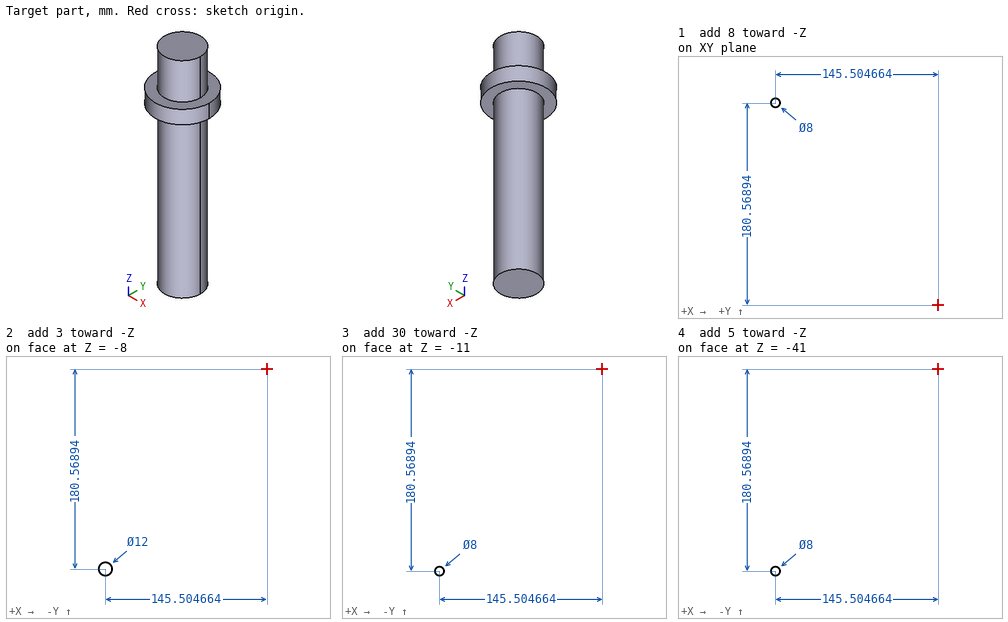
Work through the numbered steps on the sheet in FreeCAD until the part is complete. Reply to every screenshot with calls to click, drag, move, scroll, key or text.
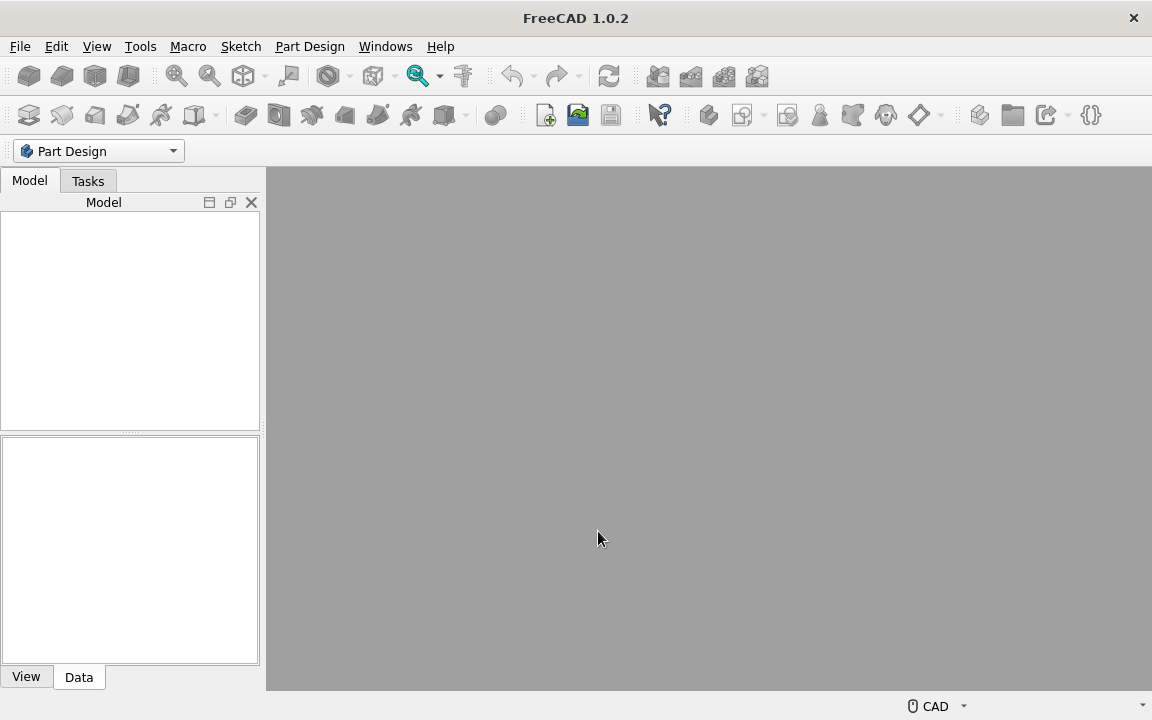
click(545, 116)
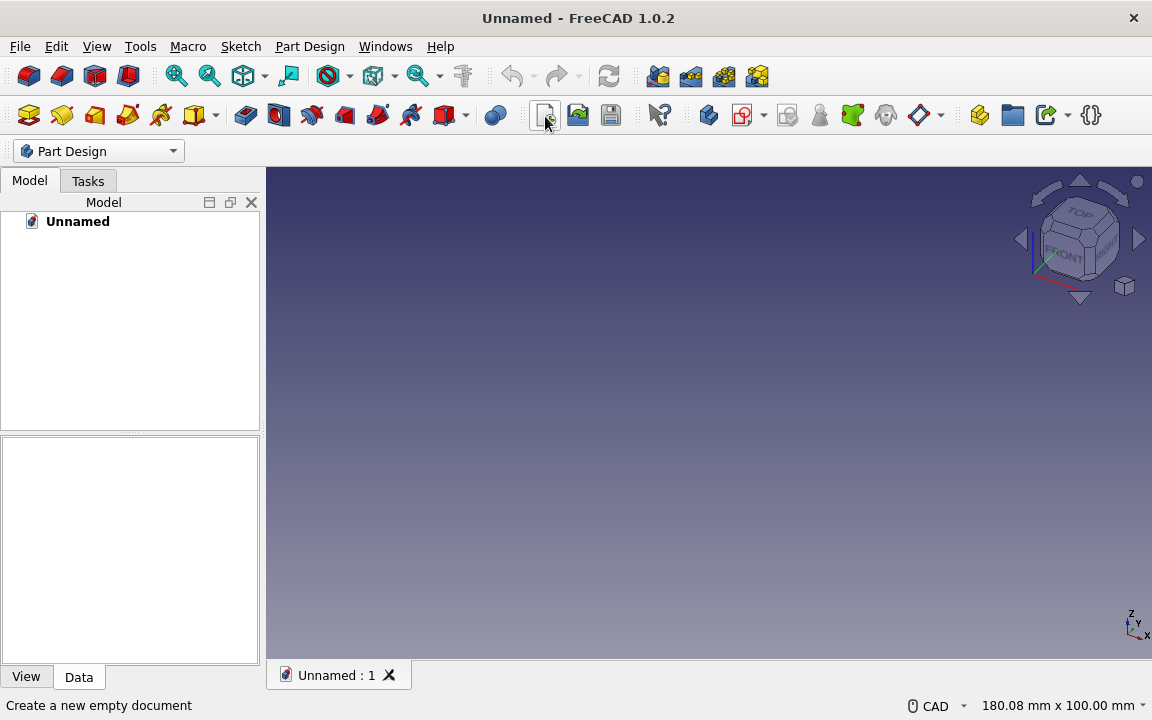
click(742, 116)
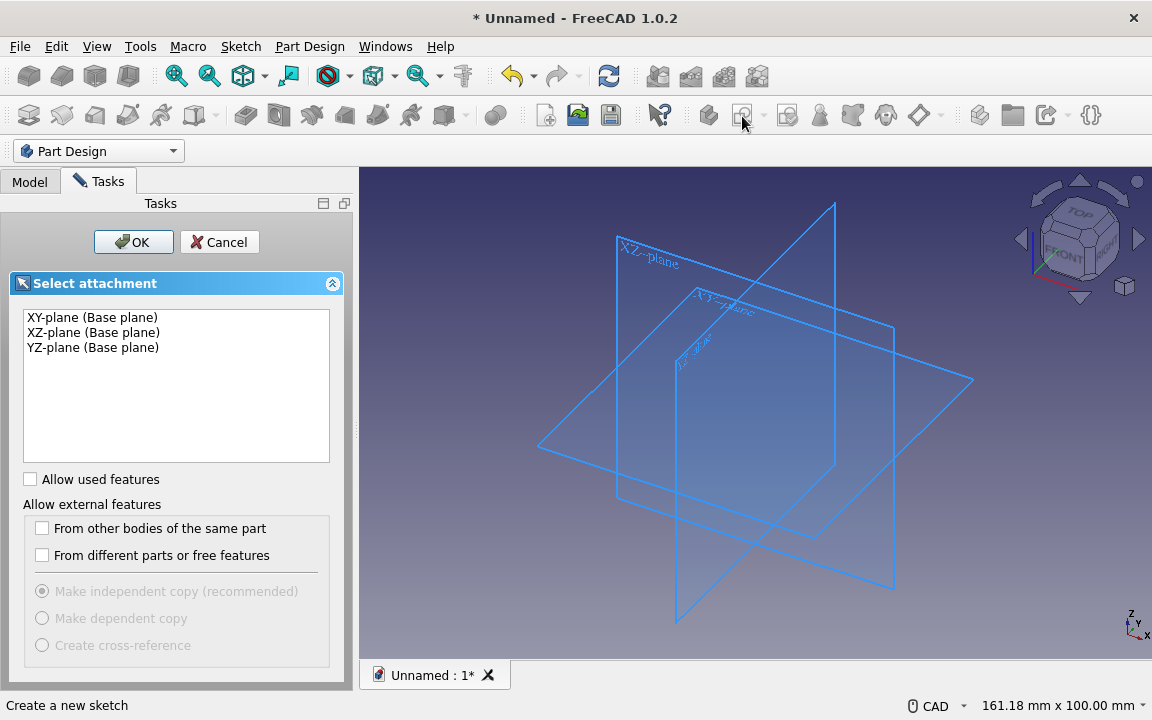
click(84, 318)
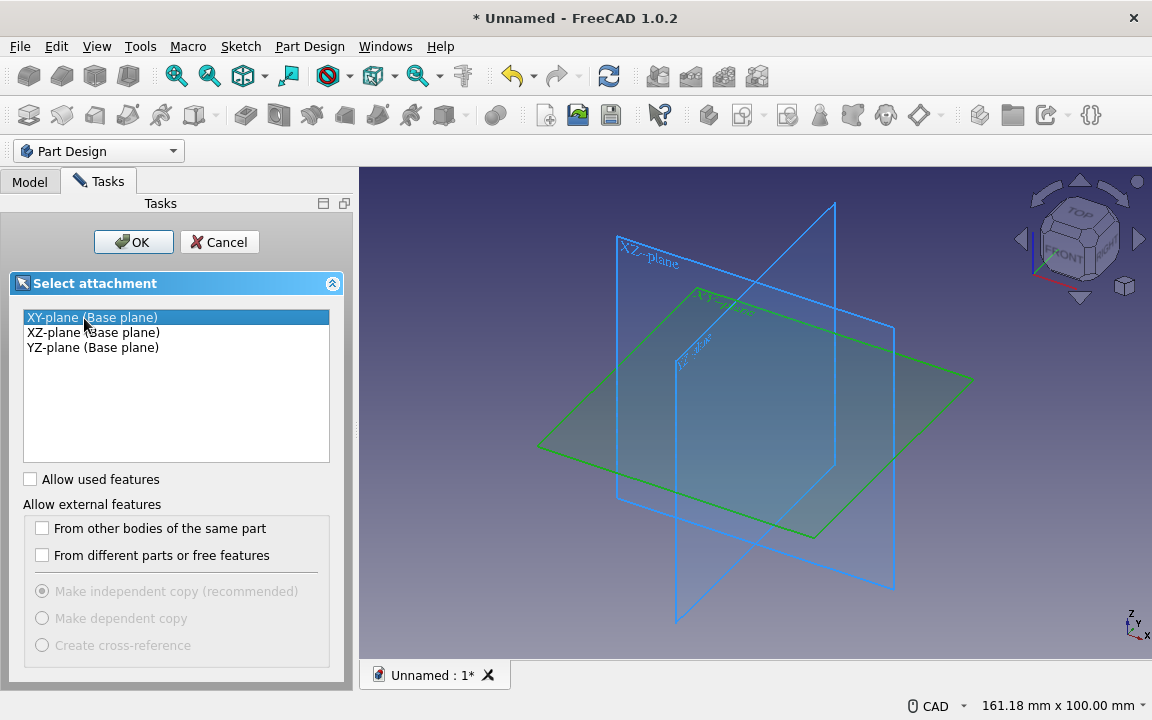
click(134, 242)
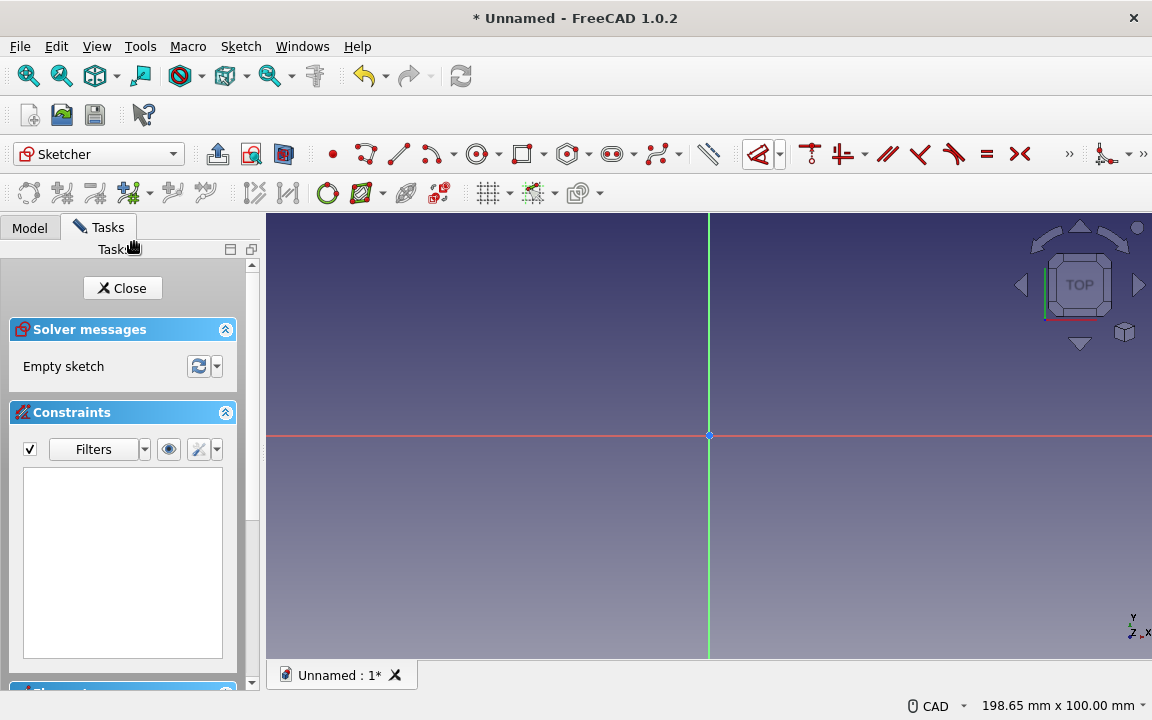
scroll(640, 436, down, 5)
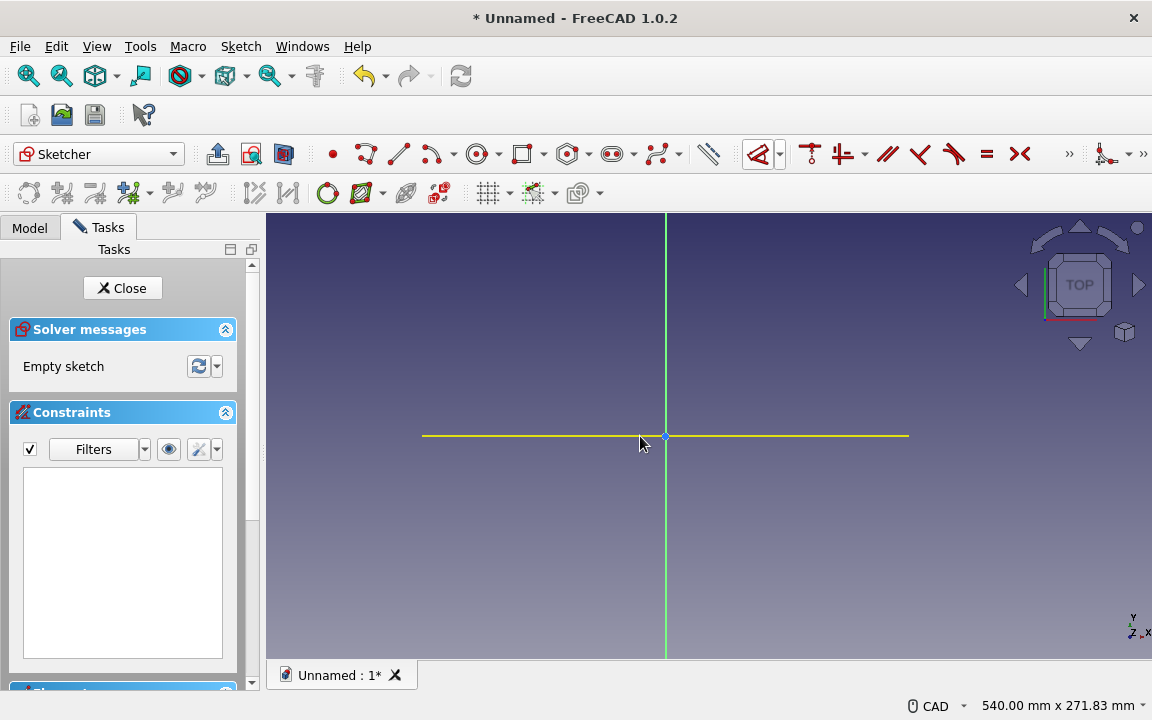
scroll(640, 436, down, 5)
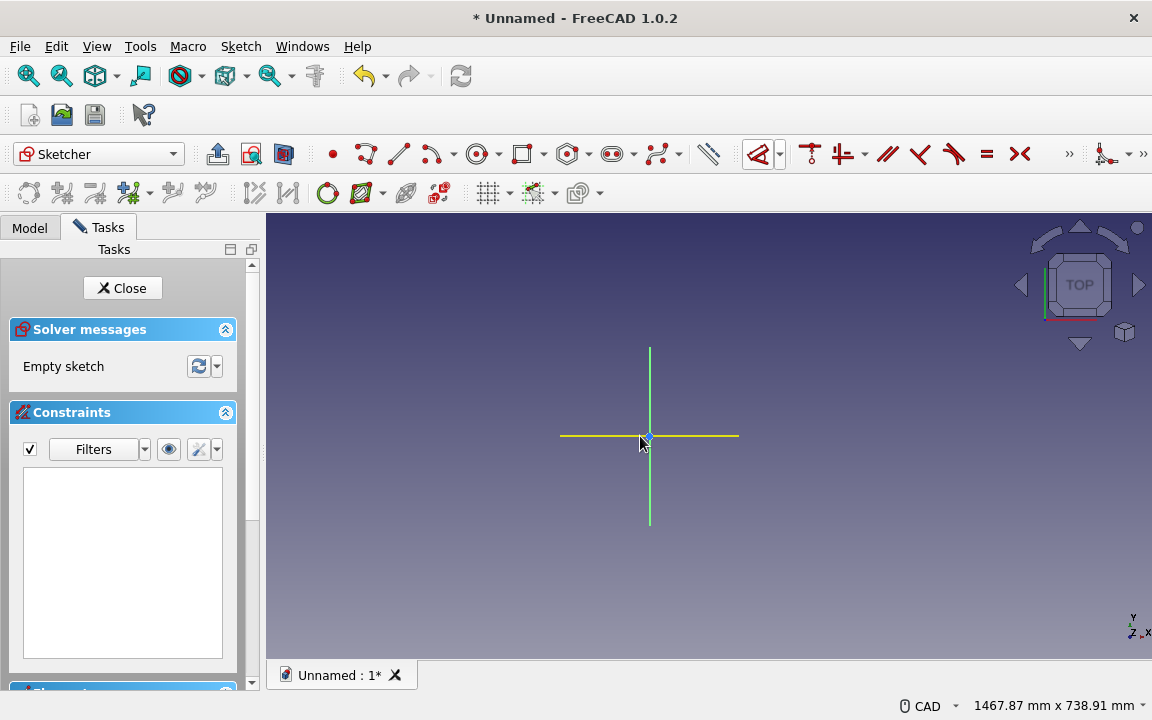
scroll(558, 322, up, 15)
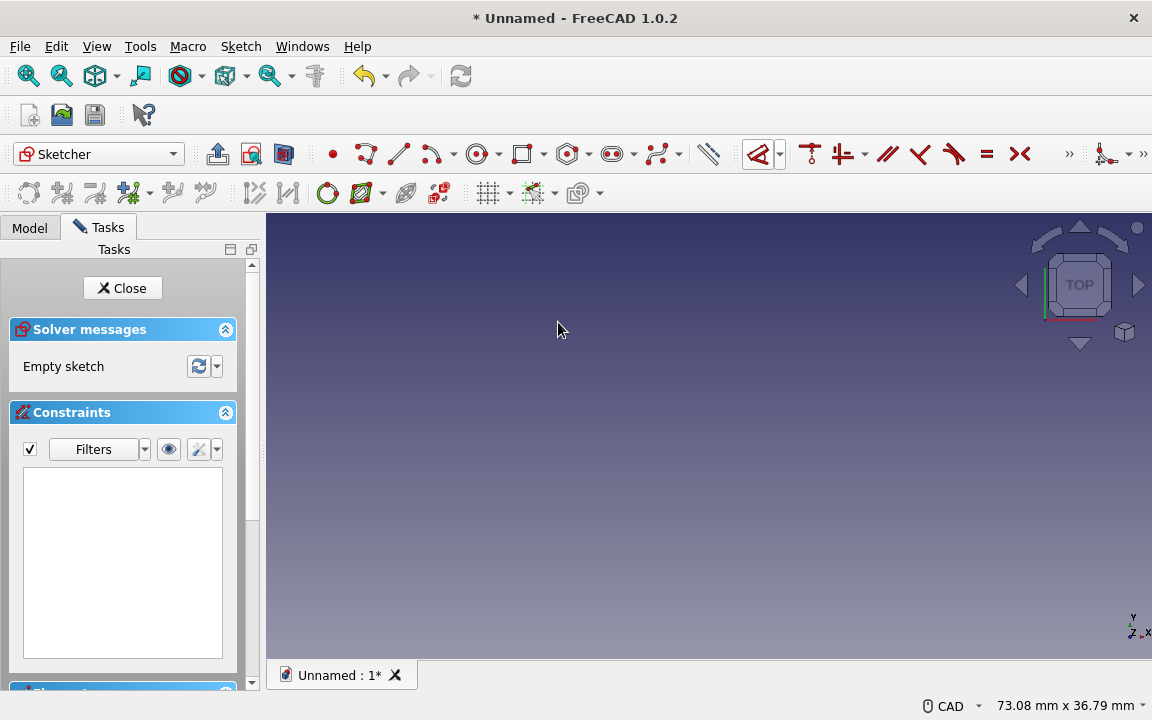
scroll(623, 421, up, 5)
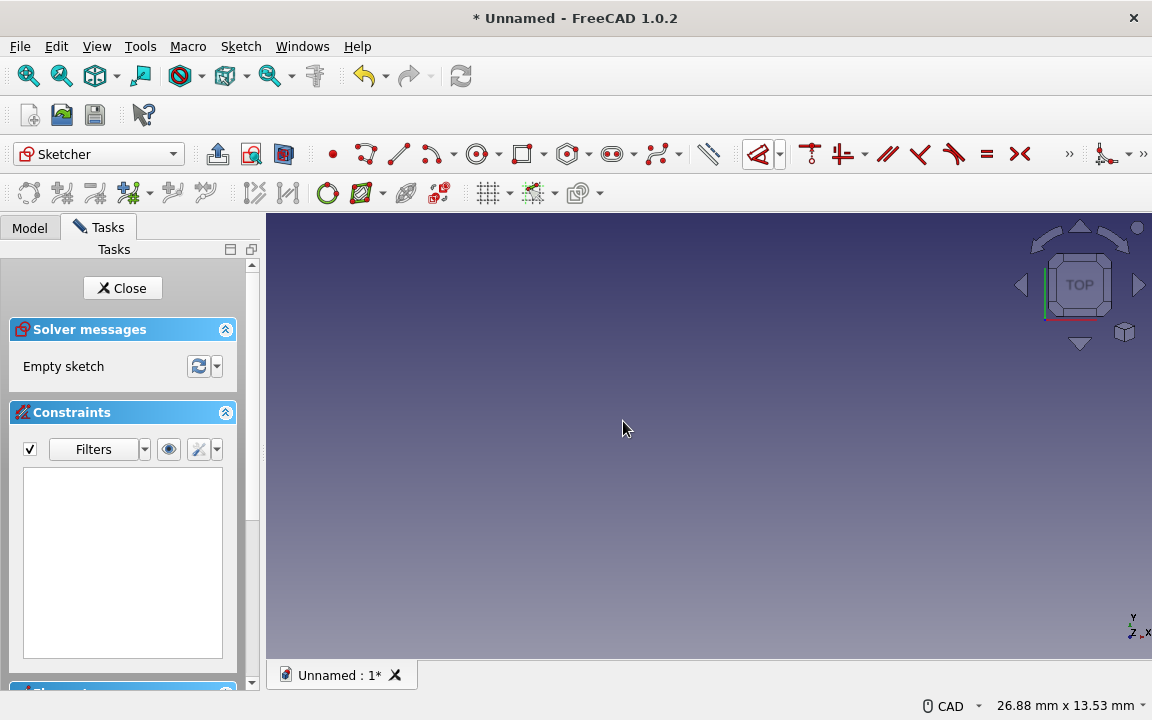
click(476, 154)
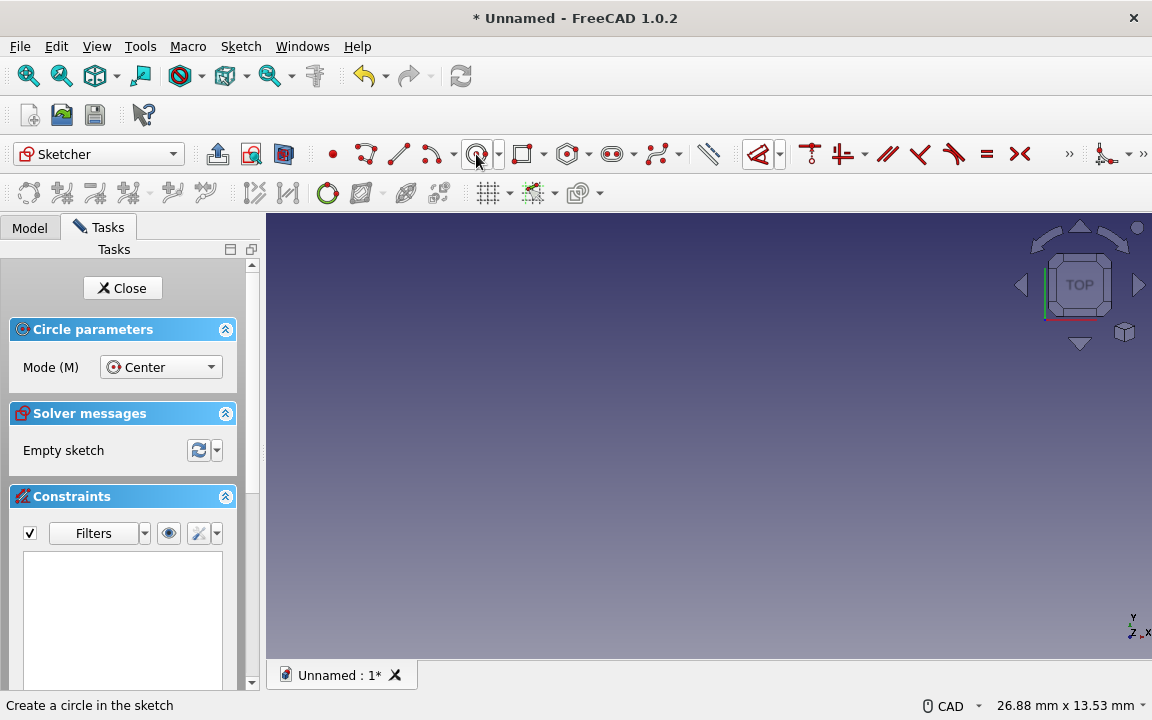
click(640, 436)
click(733, 342)
key(Escape)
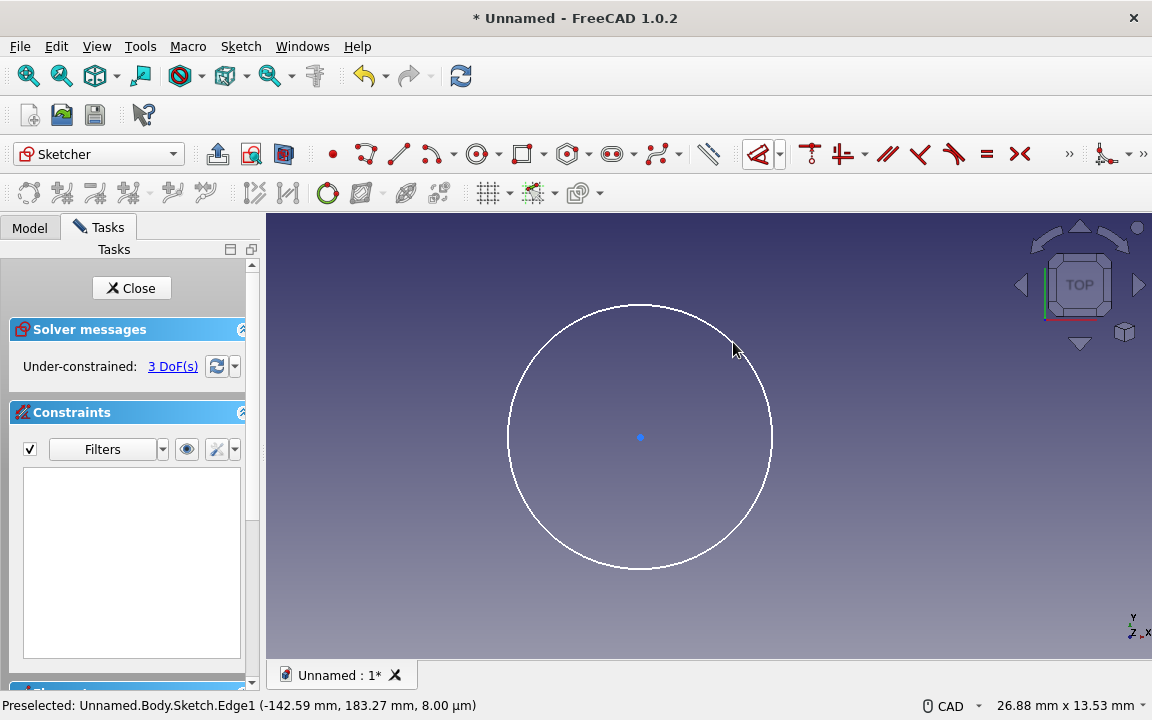
click(733, 343)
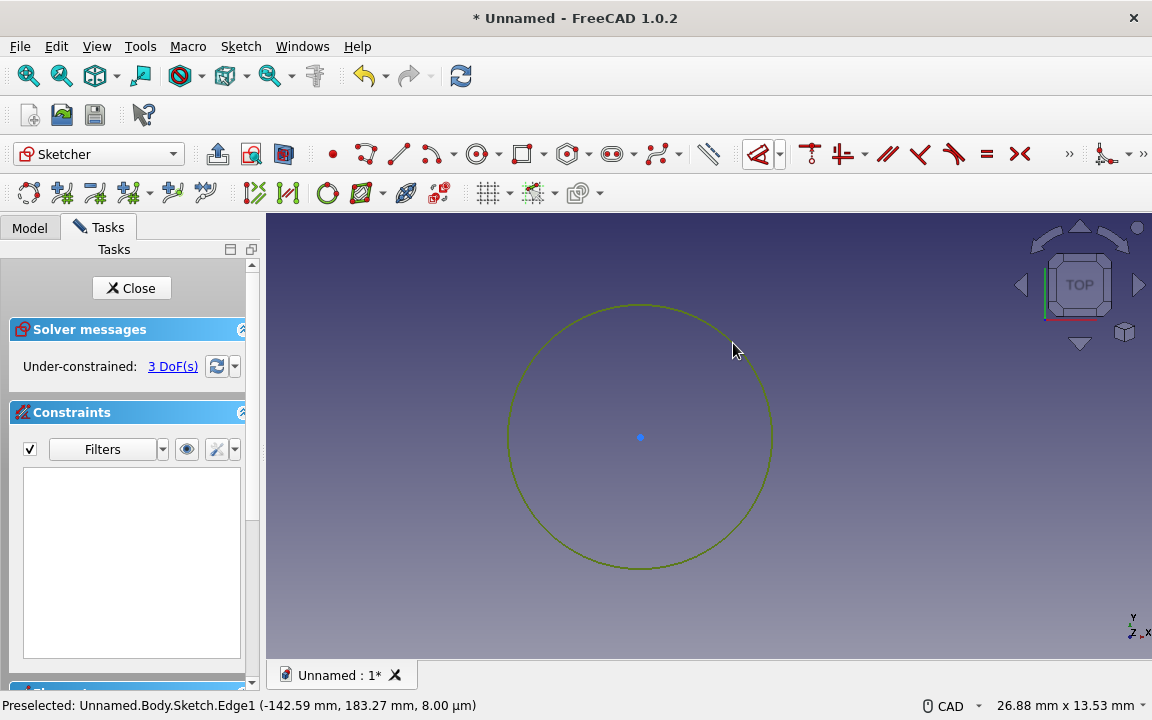
click(780, 154)